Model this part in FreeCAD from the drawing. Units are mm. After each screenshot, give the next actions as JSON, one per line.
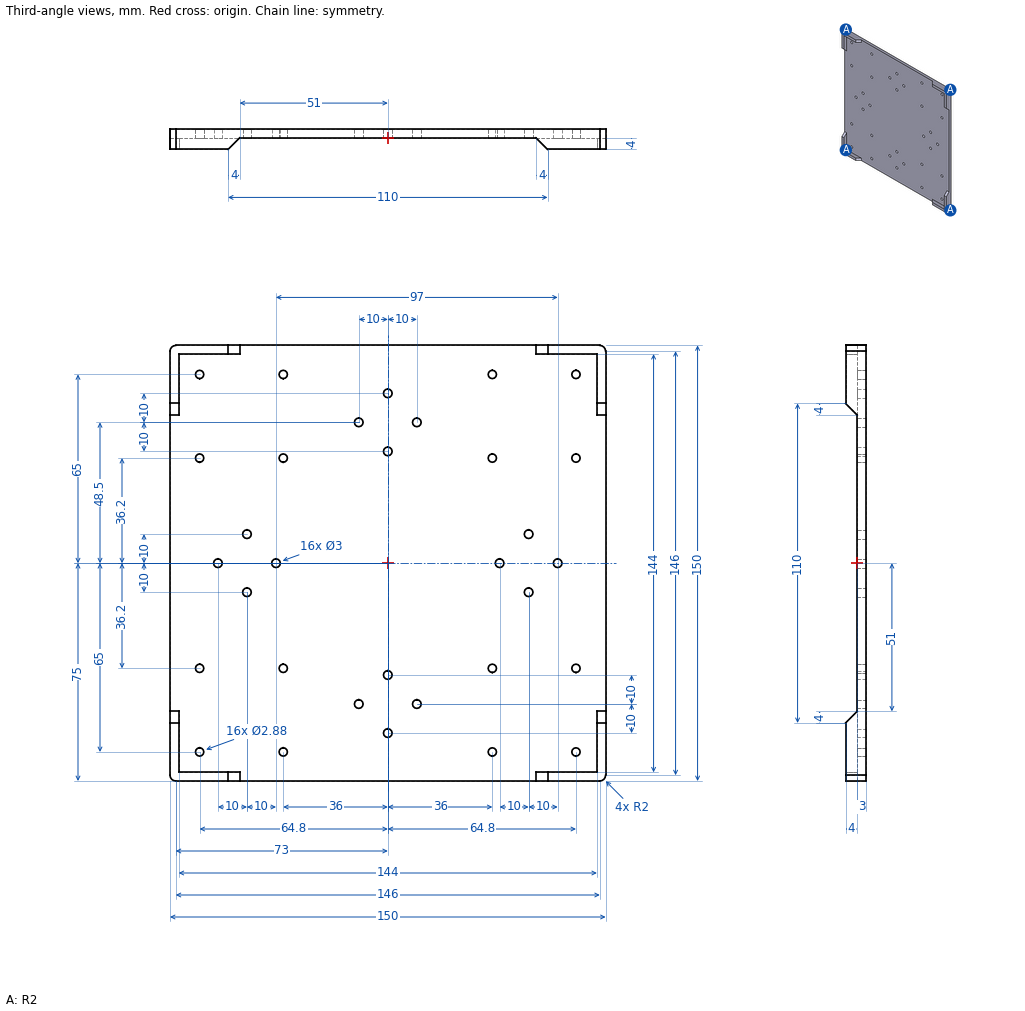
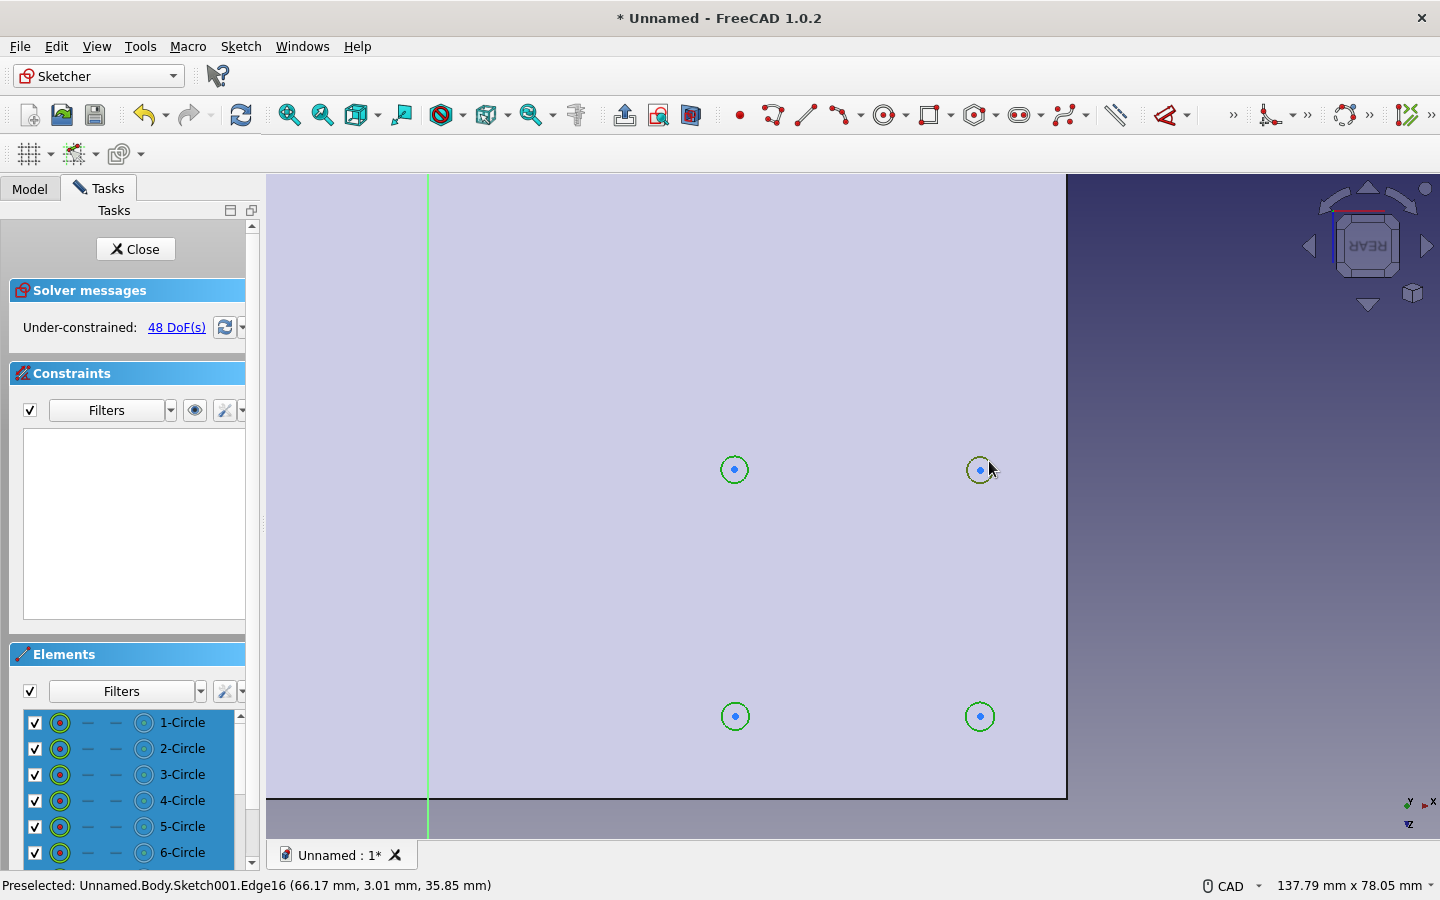
{"action": "key", "text": "e"}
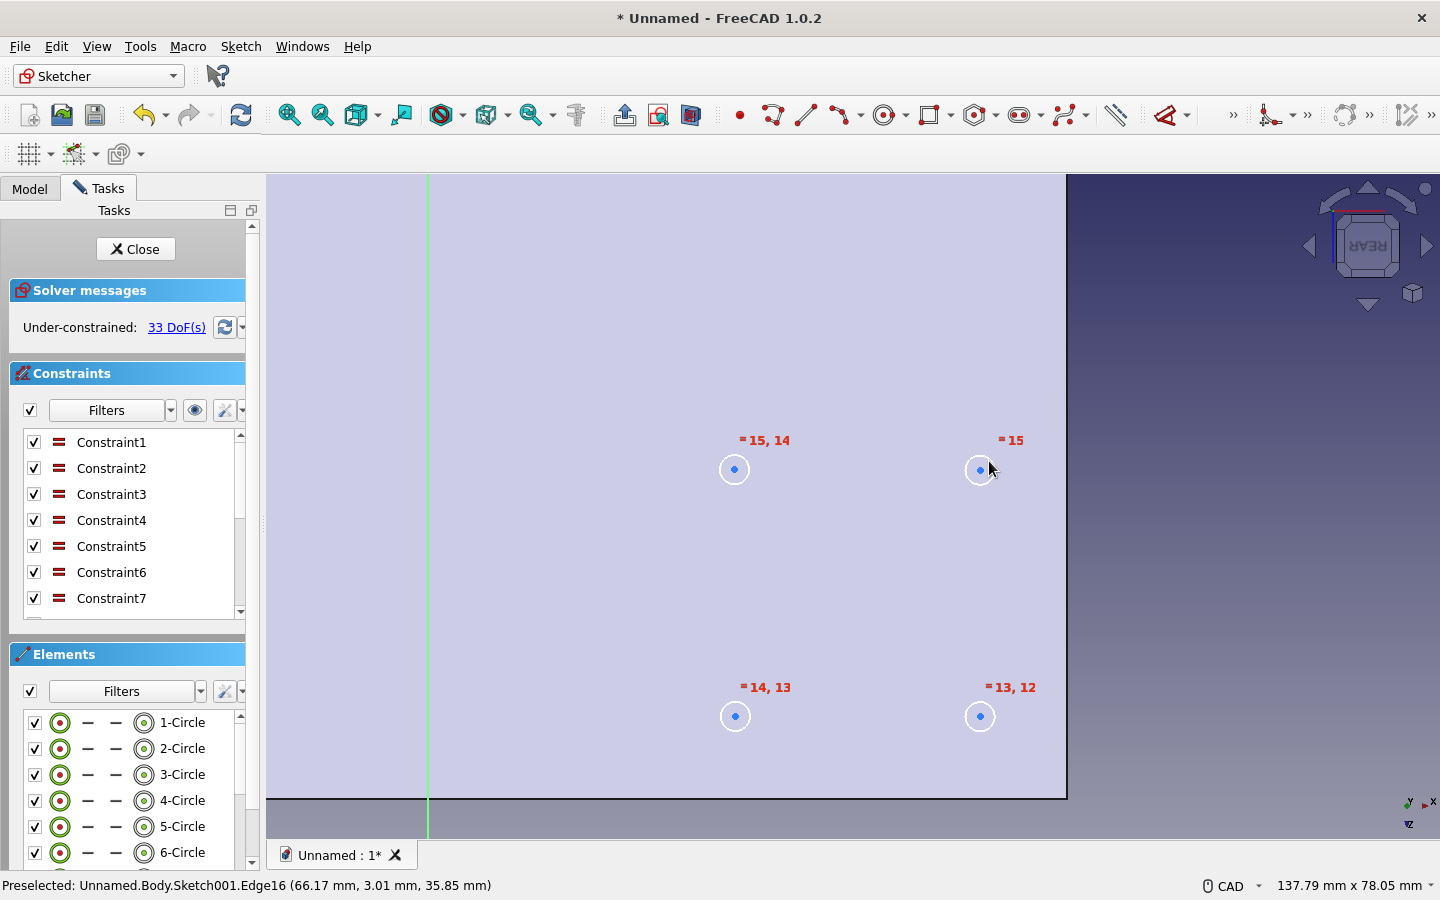
{"action": "scroll", "coordinate": [992, 708], "scroll_direction": "down", "scroll_amount": 5}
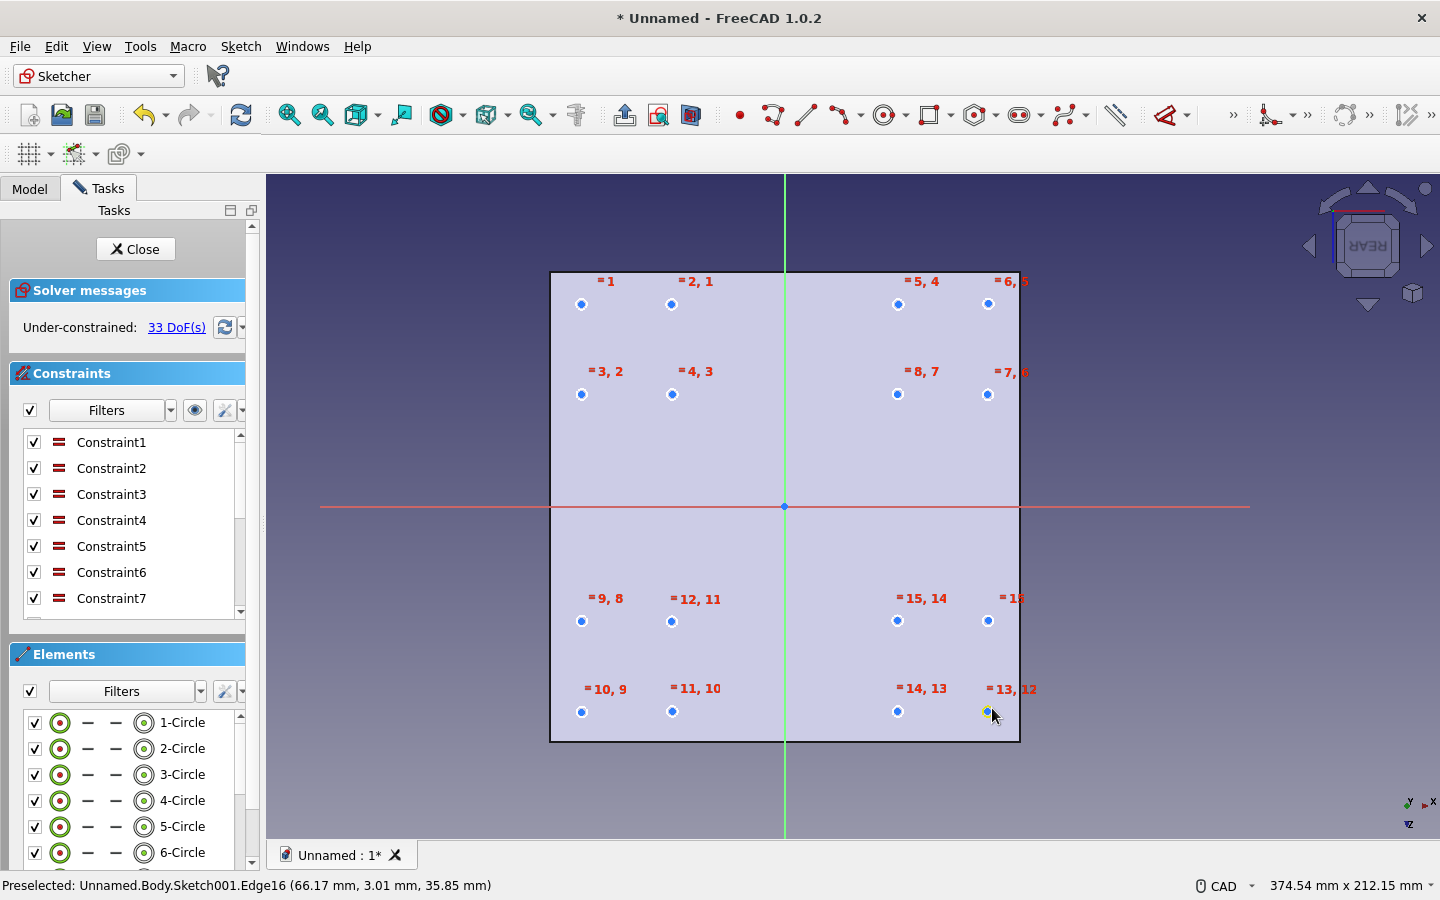
{"action": "left_click", "coordinate": [581, 304]}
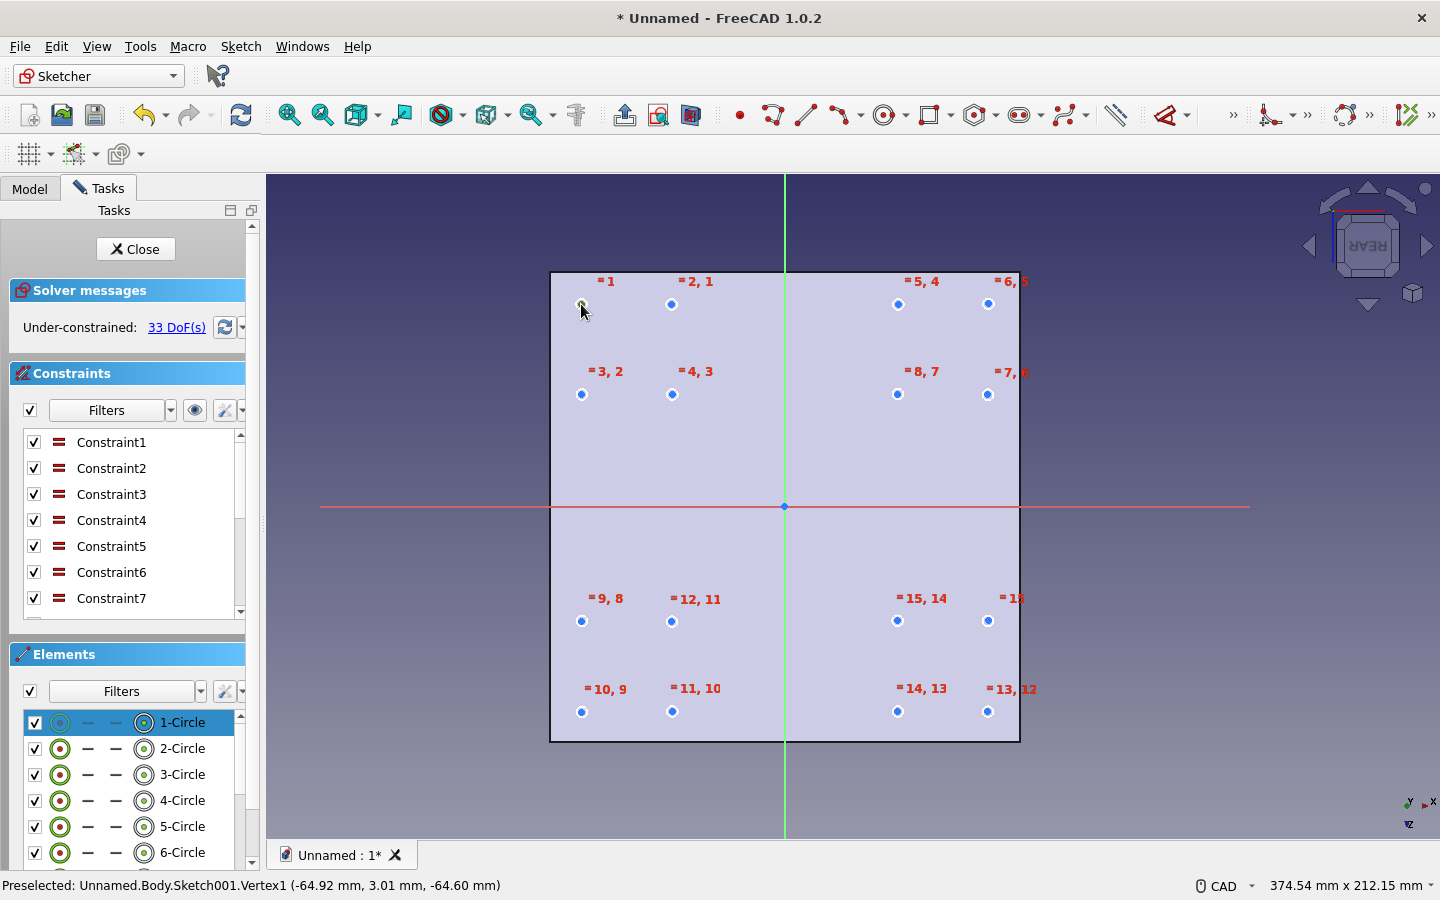
{"action": "left_click", "coordinate": [672, 304]}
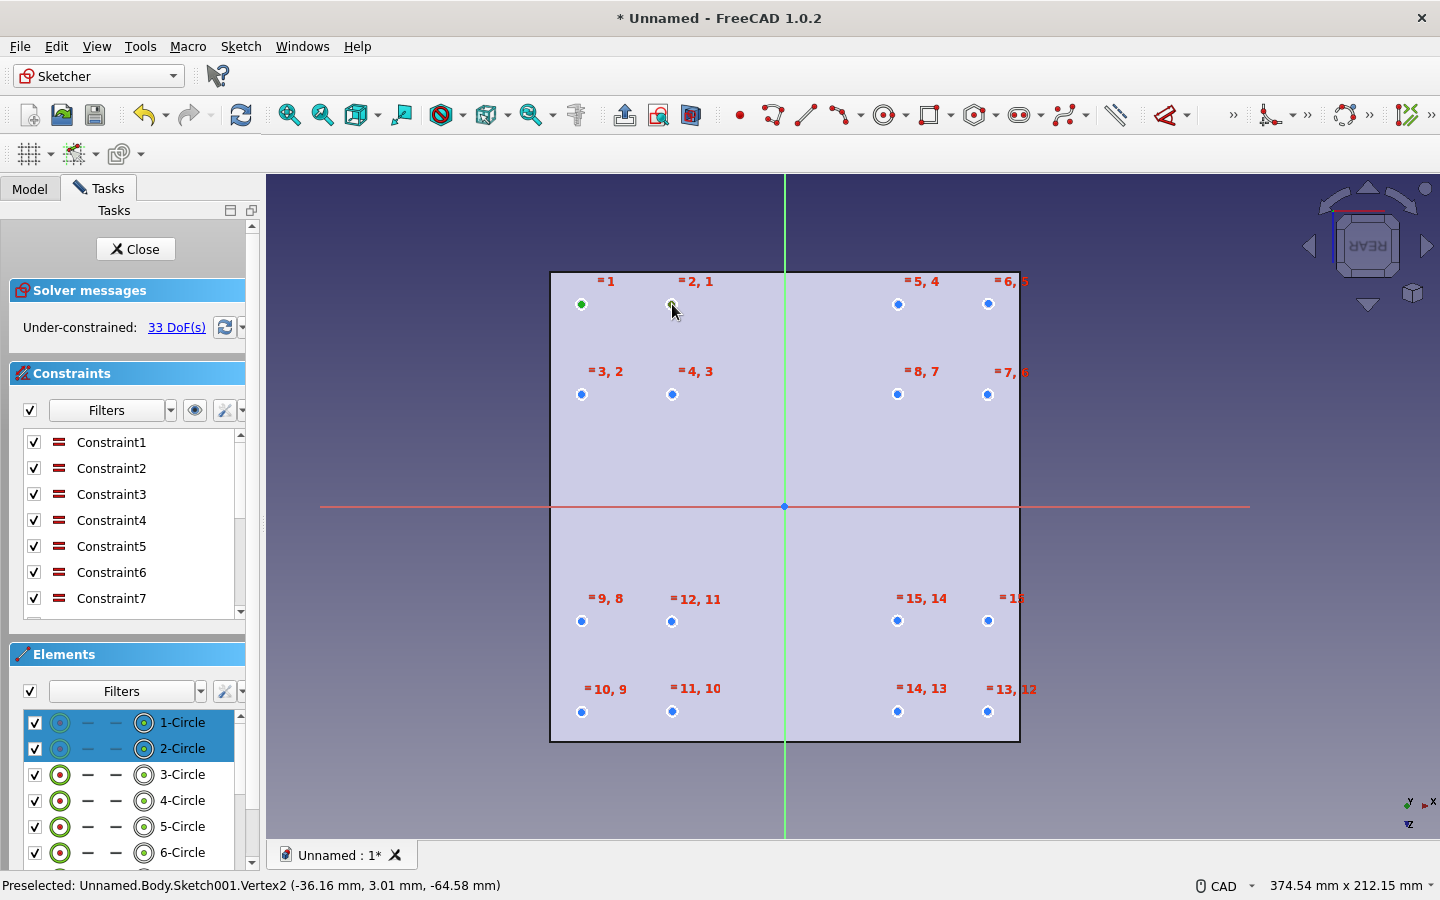
{"action": "key", "text": "h"}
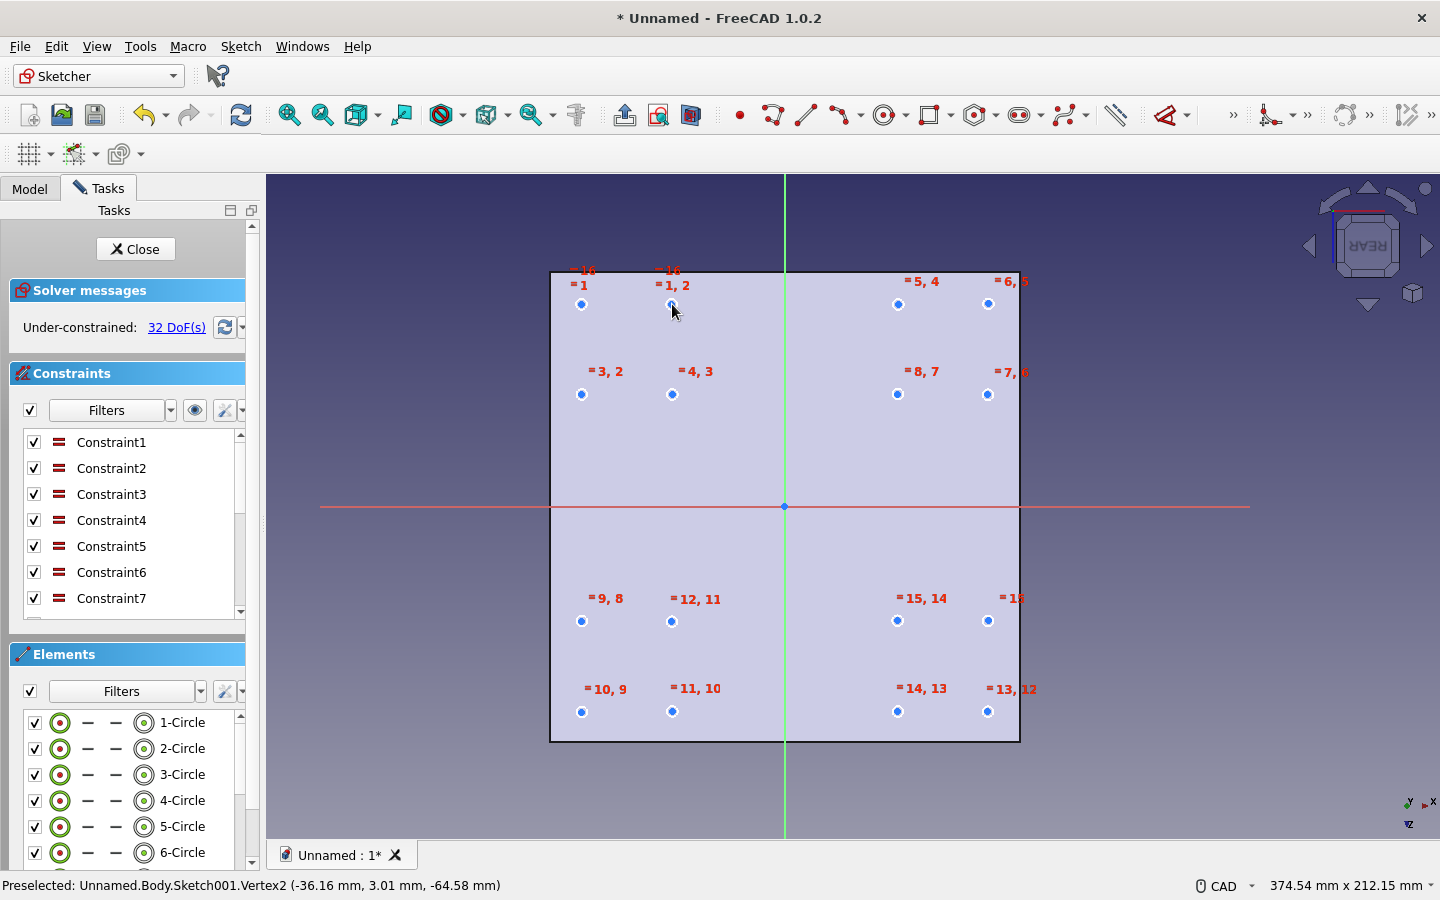
{"action": "left_click", "coordinate": [581, 304]}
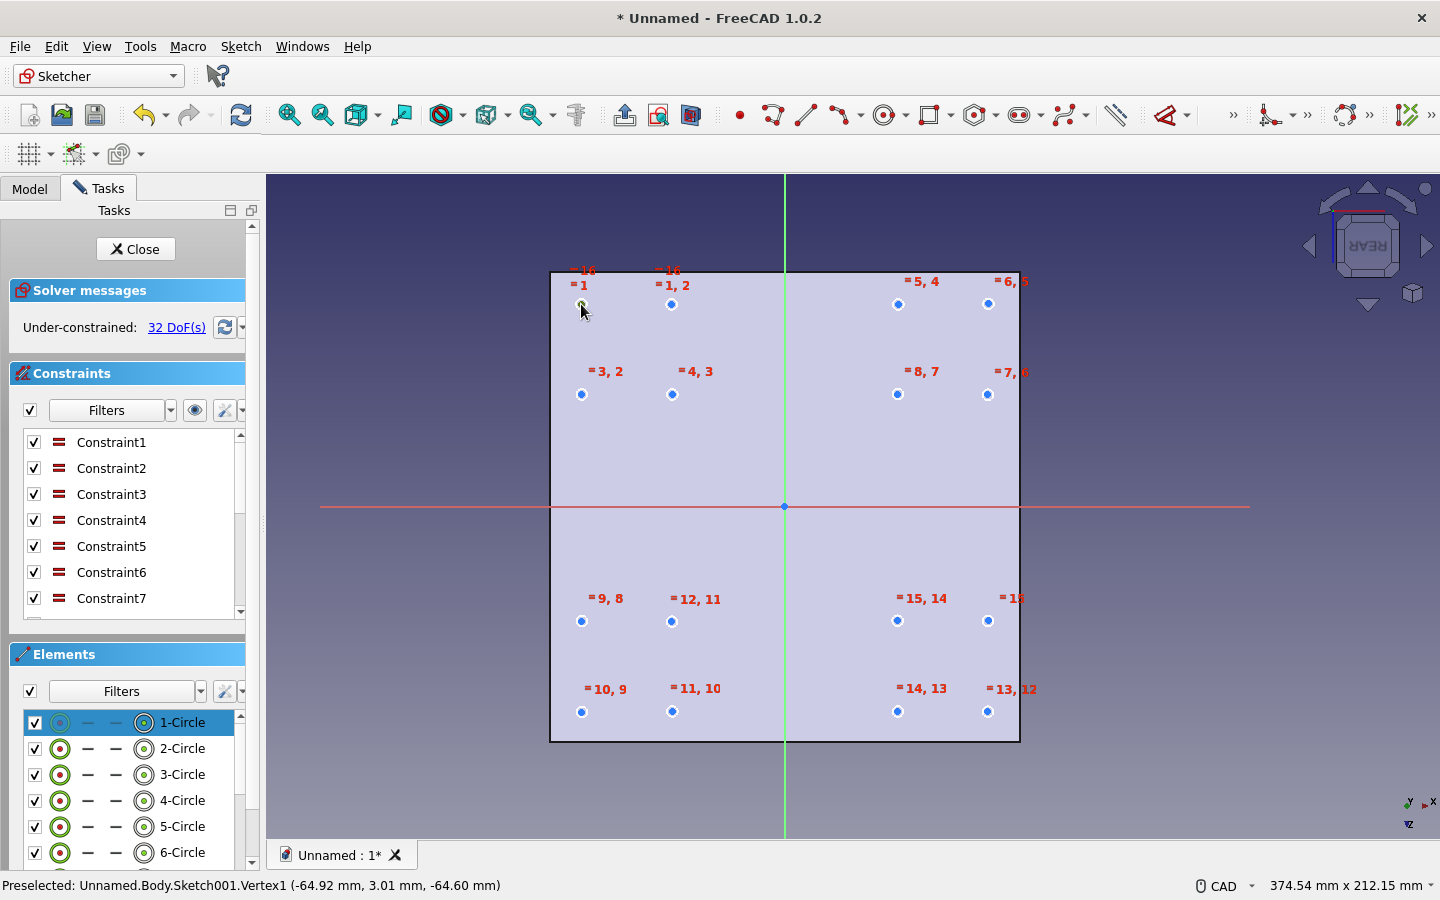
{"action": "left_click", "coordinate": [582, 394]}